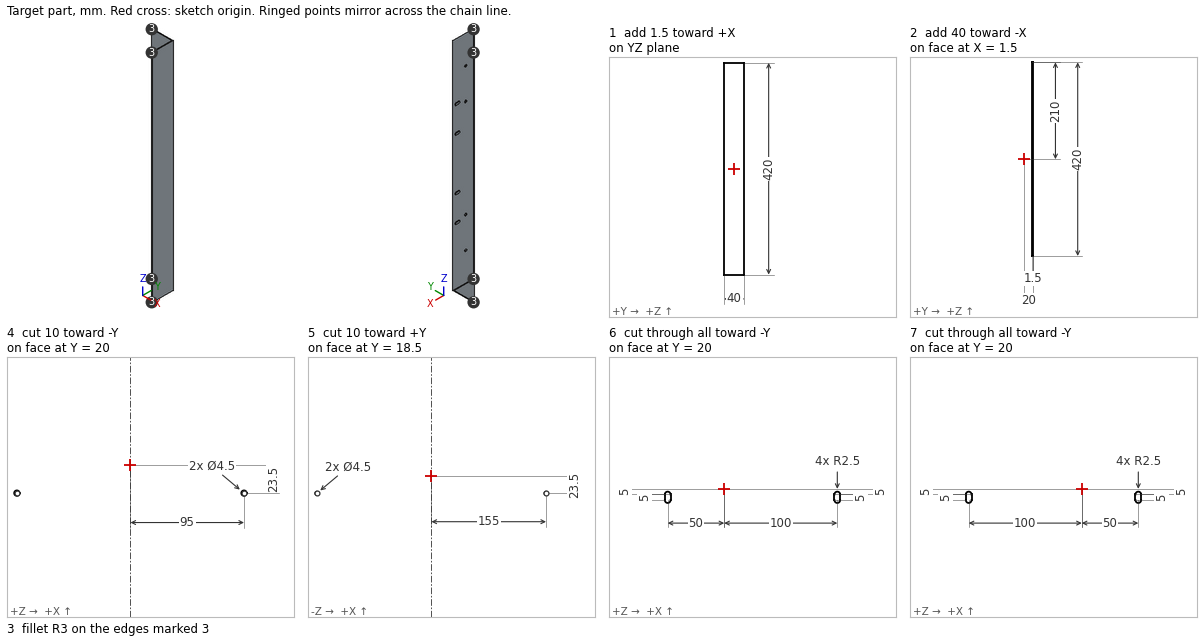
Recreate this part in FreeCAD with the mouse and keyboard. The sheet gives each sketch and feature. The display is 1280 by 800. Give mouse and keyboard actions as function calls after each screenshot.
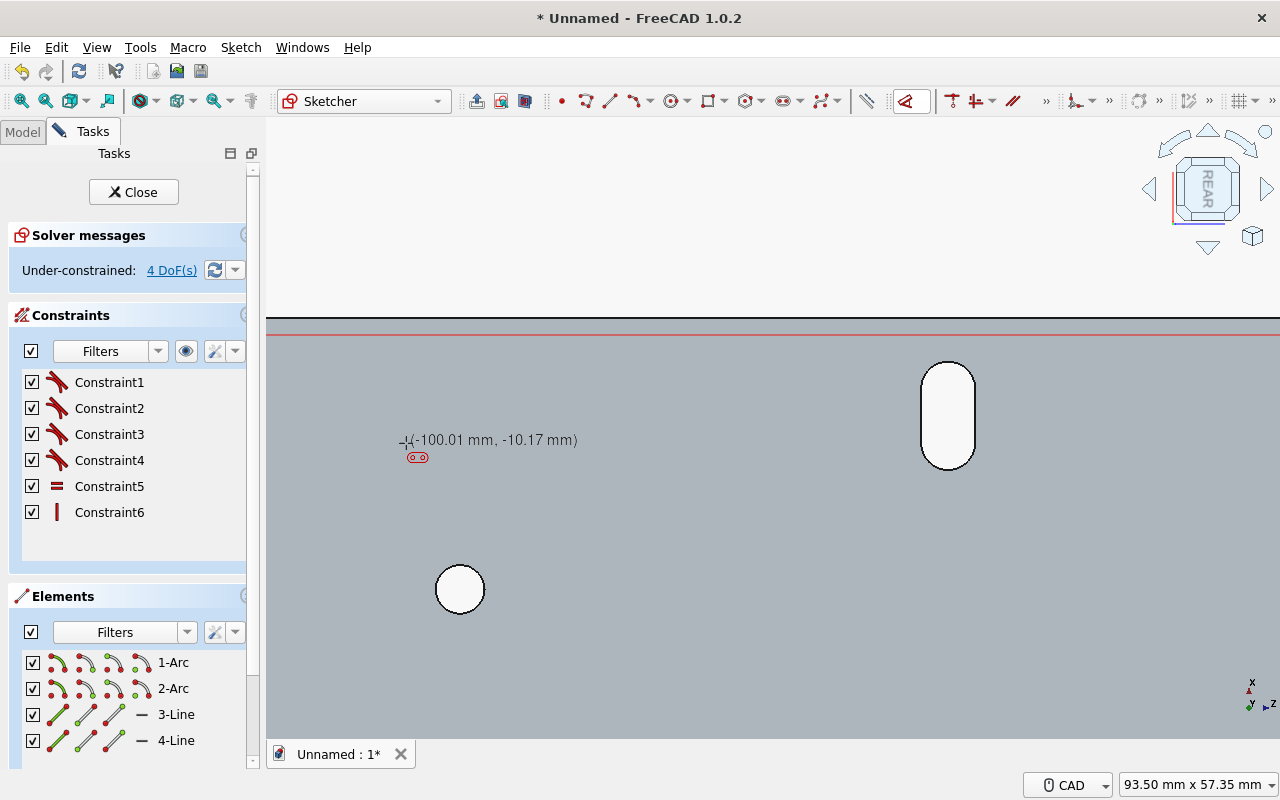
click(406, 443)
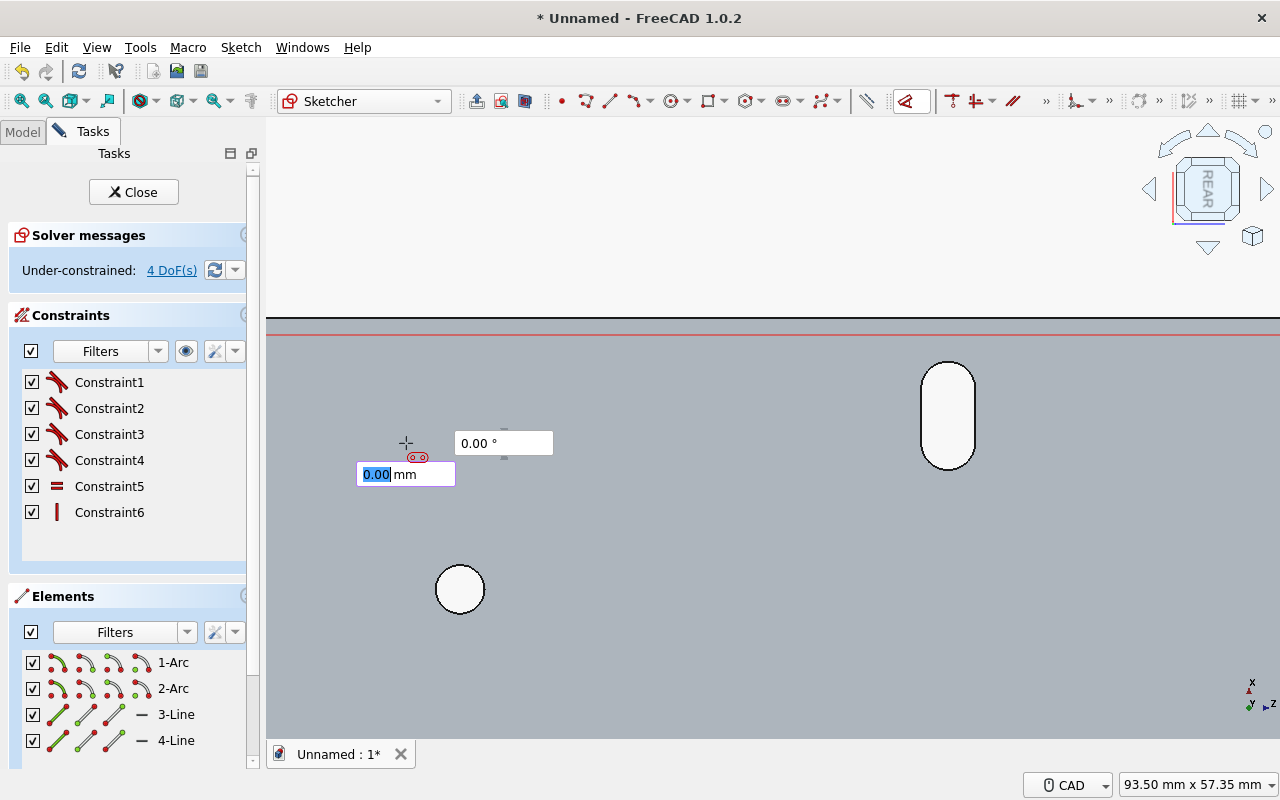
click(406, 389)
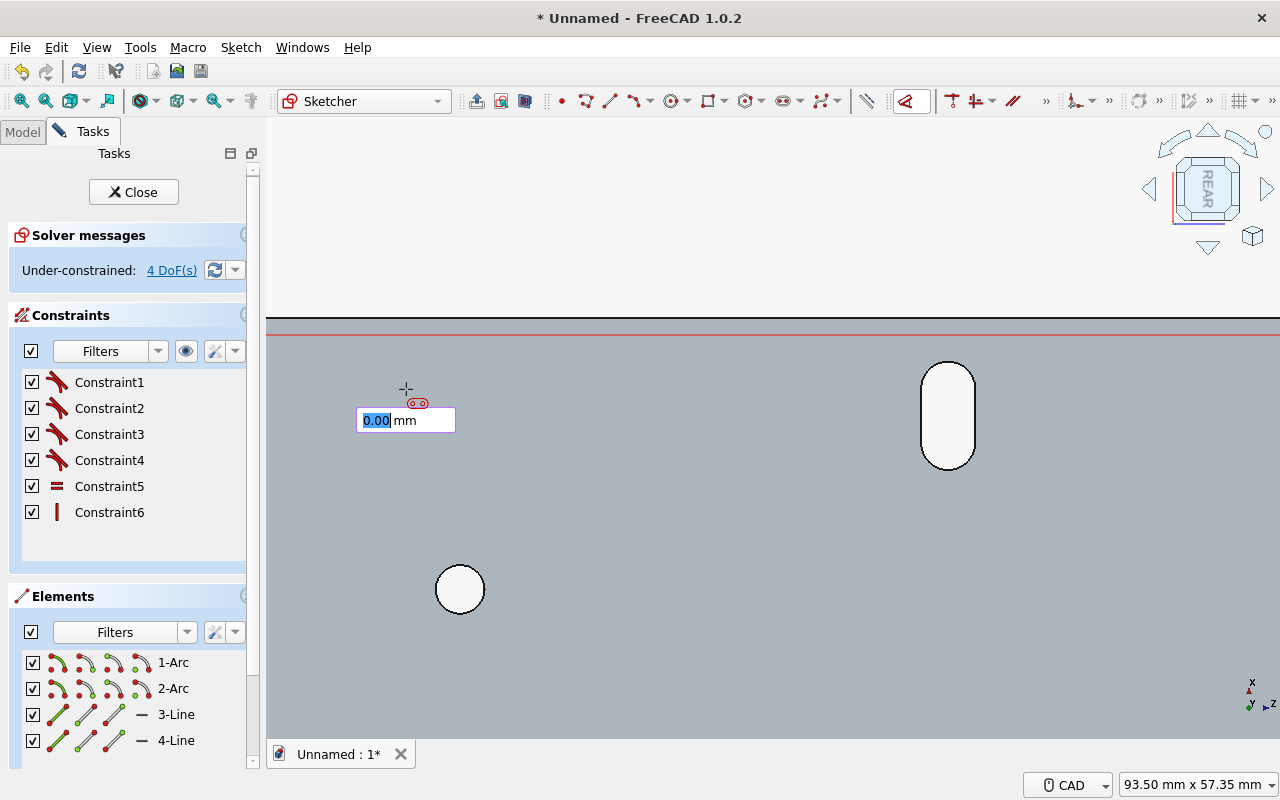
click(433, 416)
key(Escape)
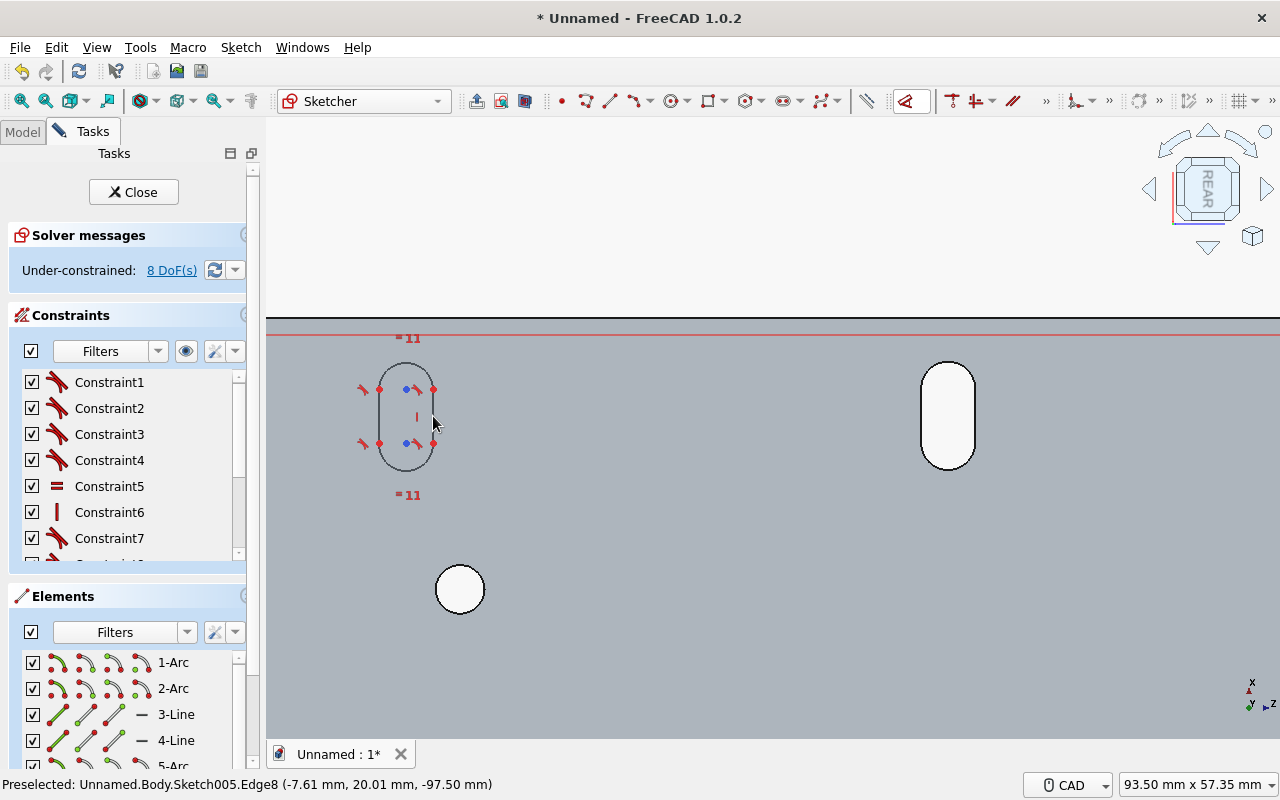
scroll(405, 443, down, 5)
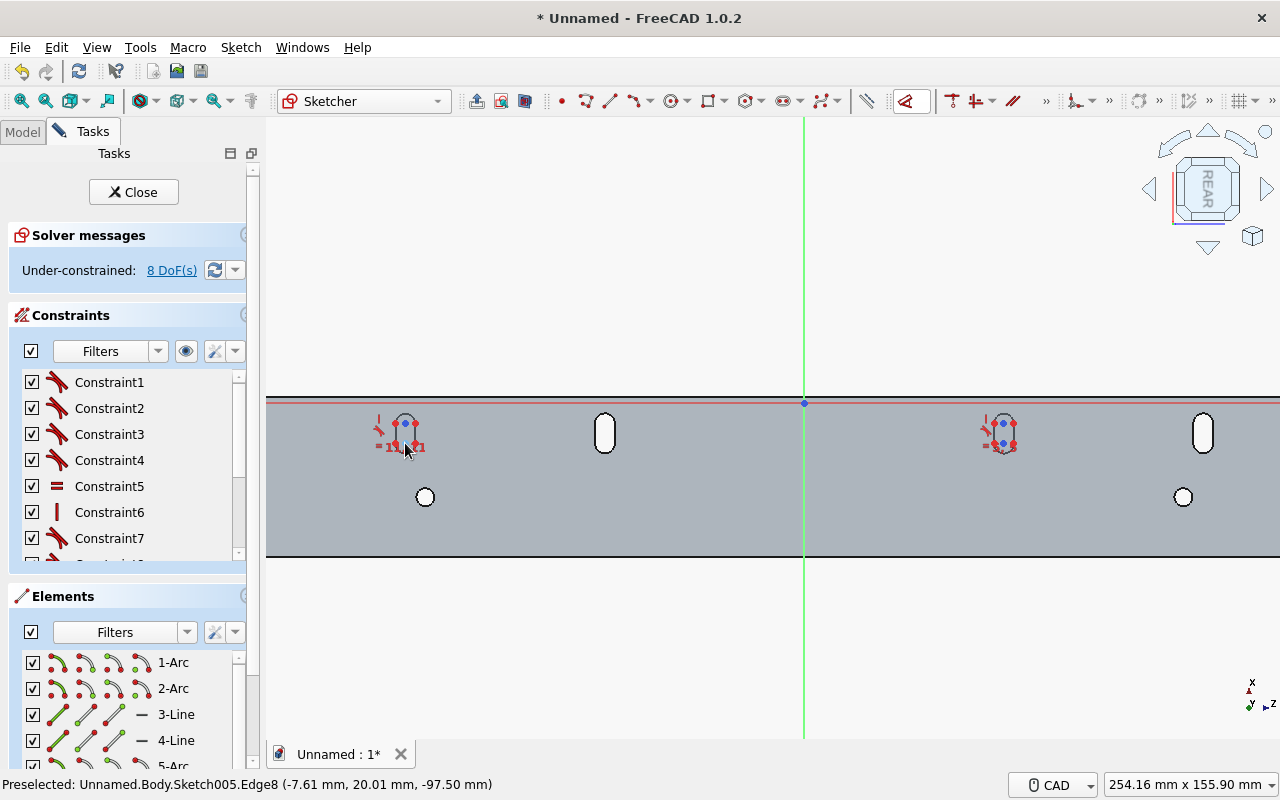
scroll(998, 452, up, 3)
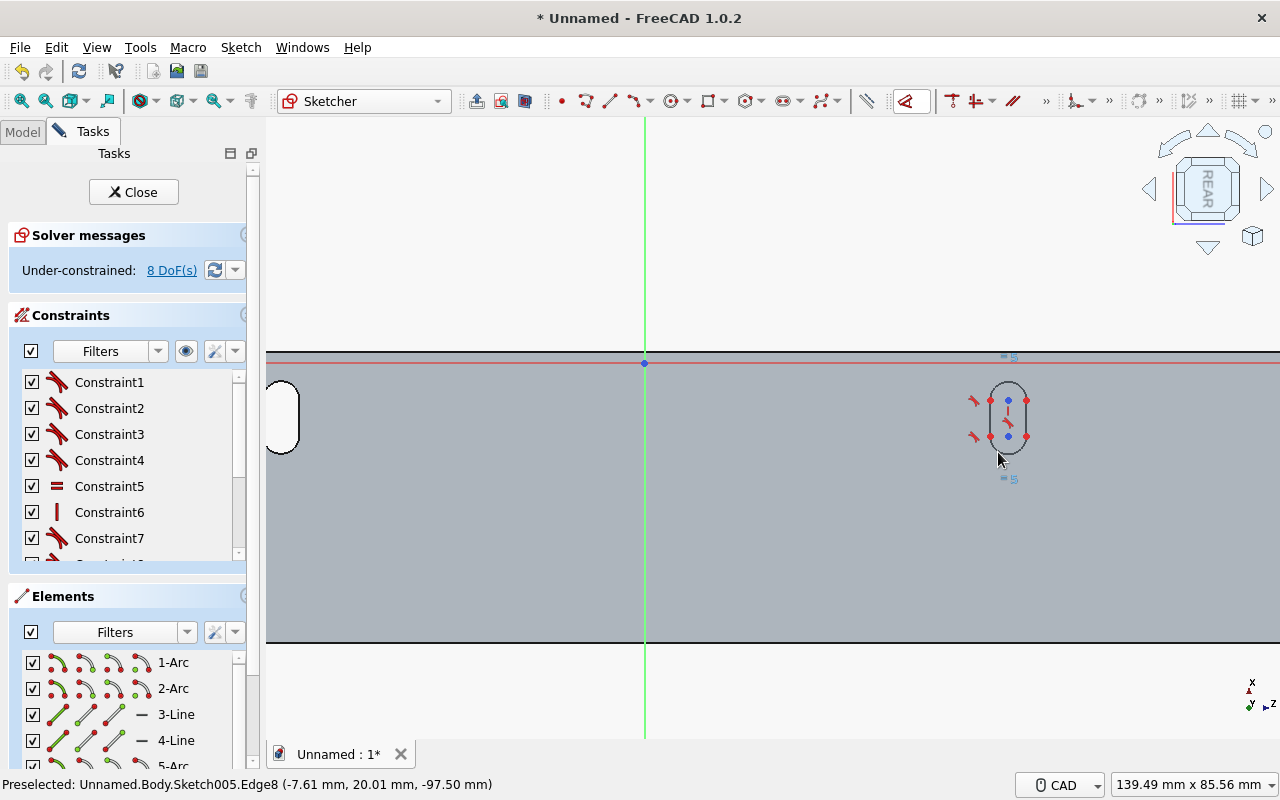
click(998, 451)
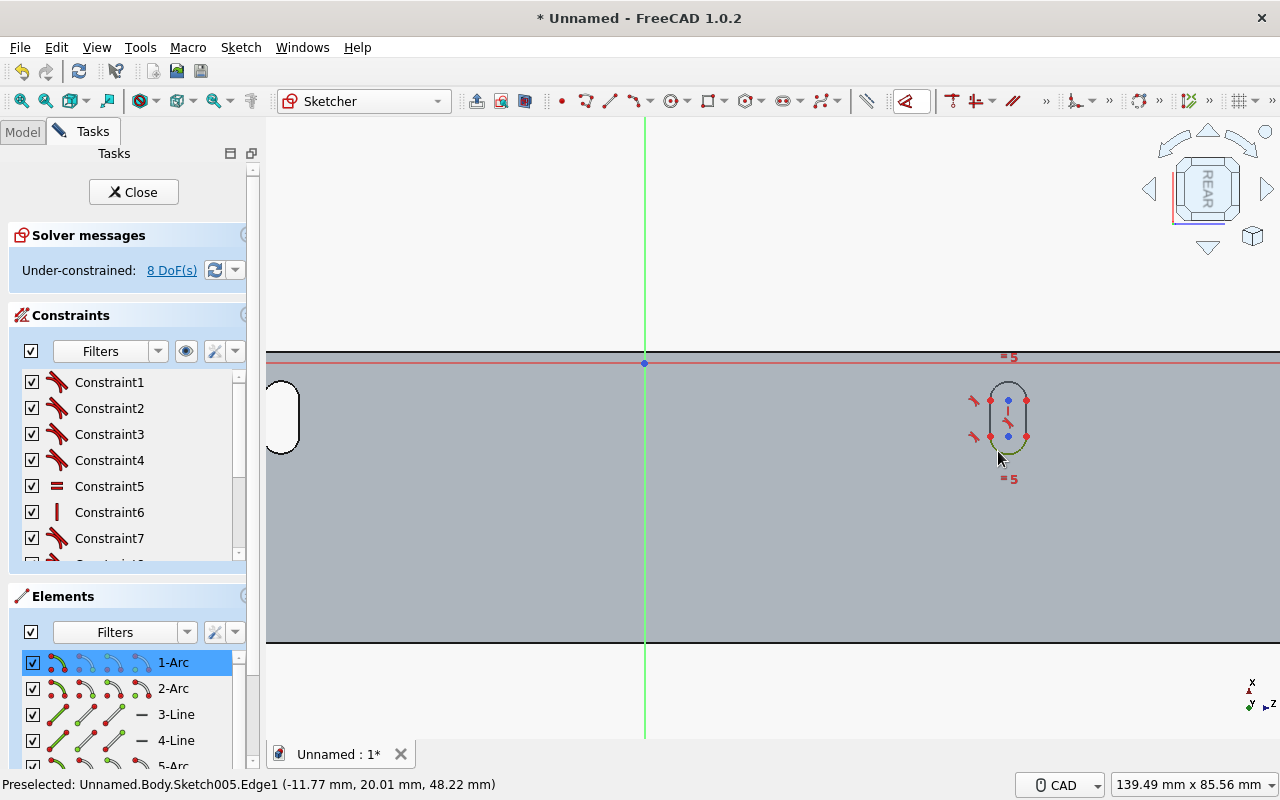
scroll(998, 452, down, 3)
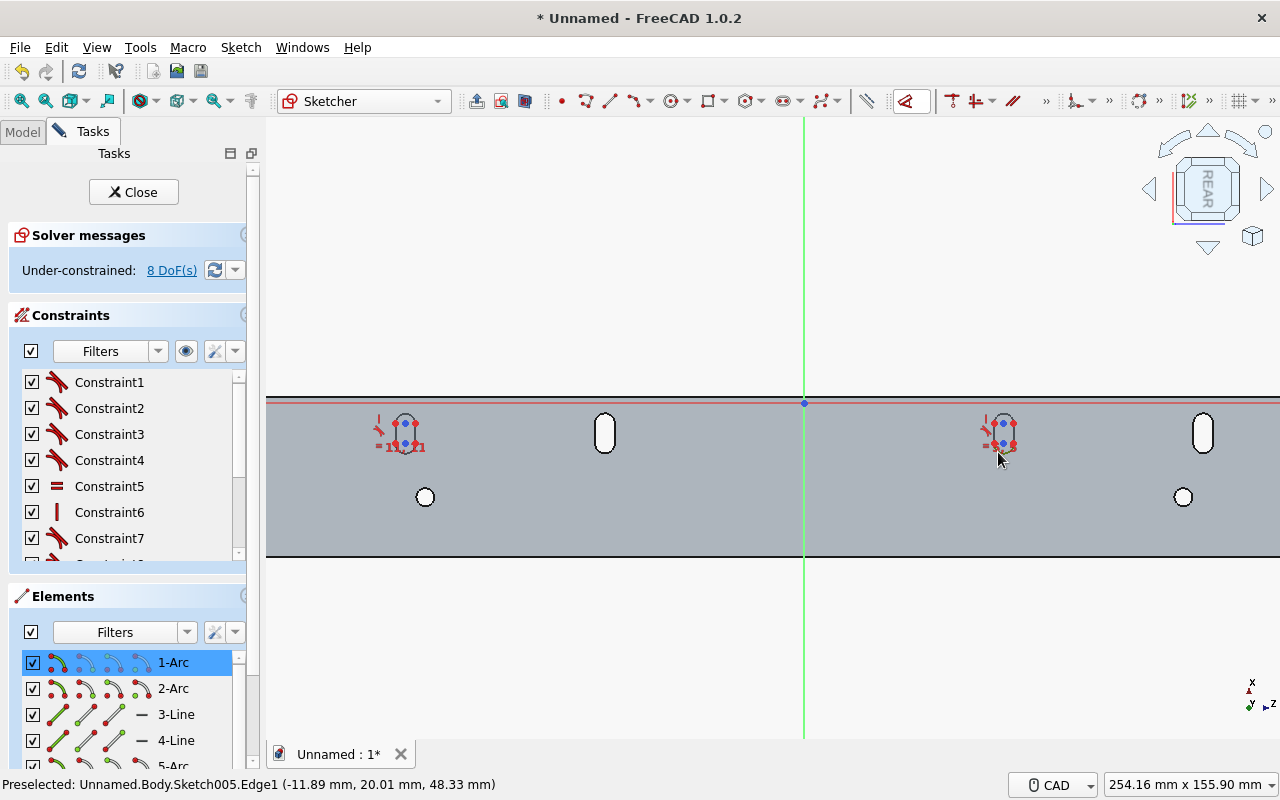
scroll(400, 452, up, 3)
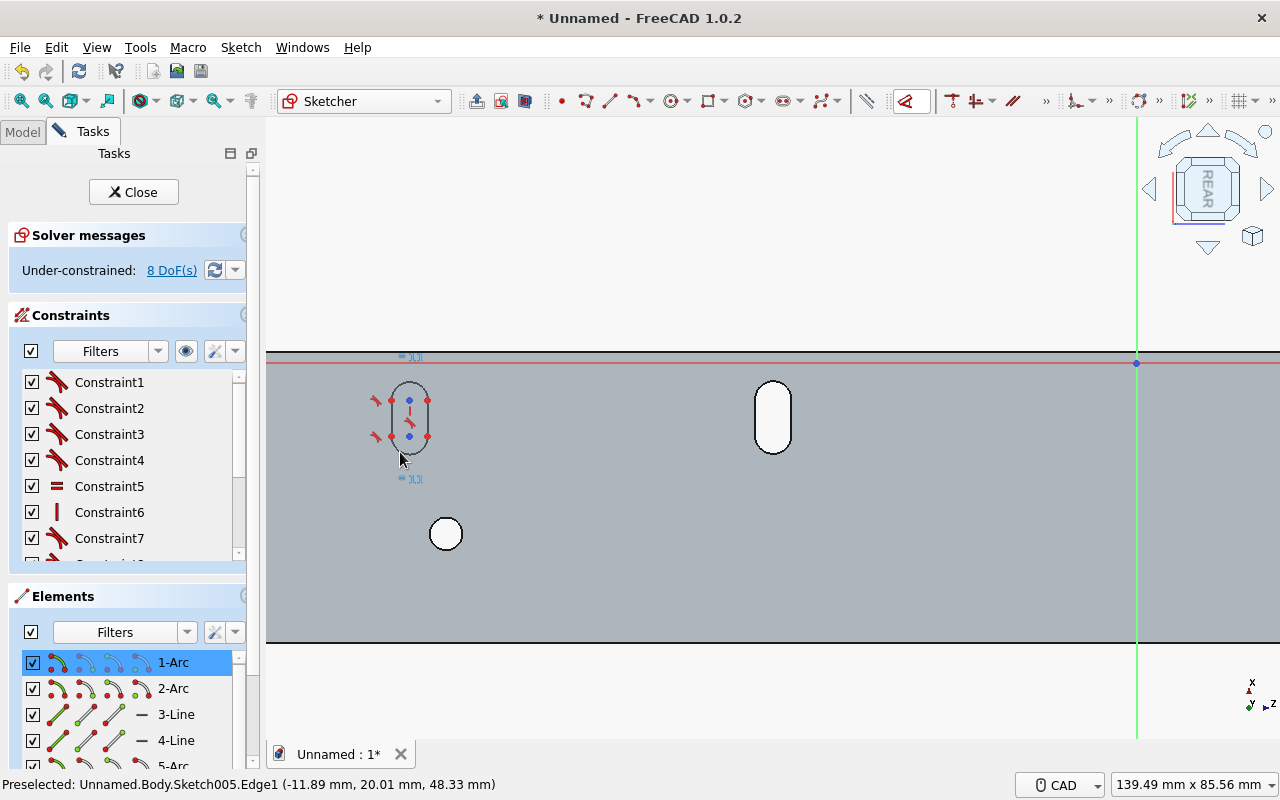
click(399, 451)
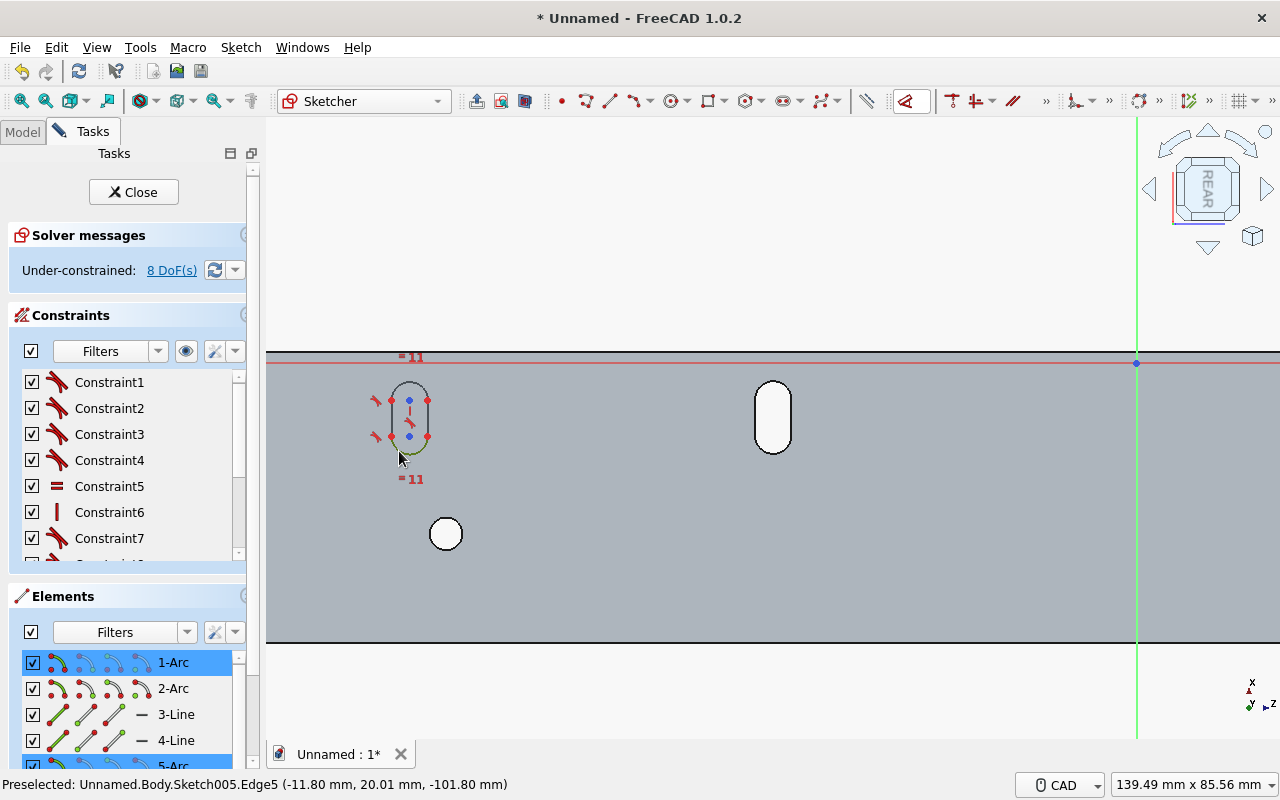
key(e)